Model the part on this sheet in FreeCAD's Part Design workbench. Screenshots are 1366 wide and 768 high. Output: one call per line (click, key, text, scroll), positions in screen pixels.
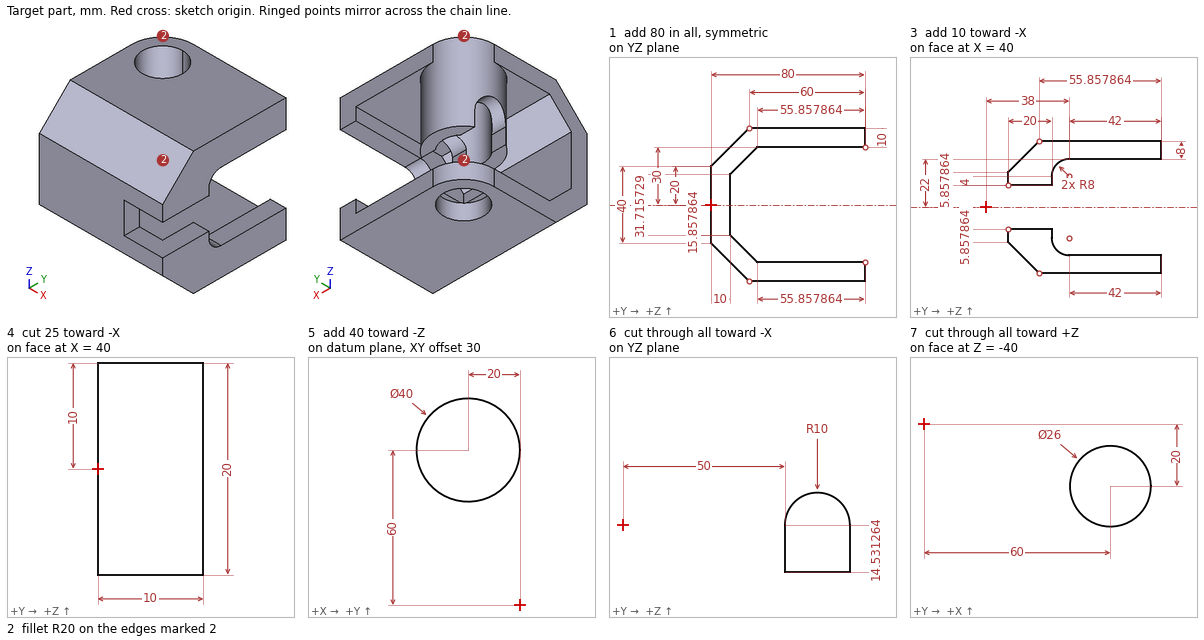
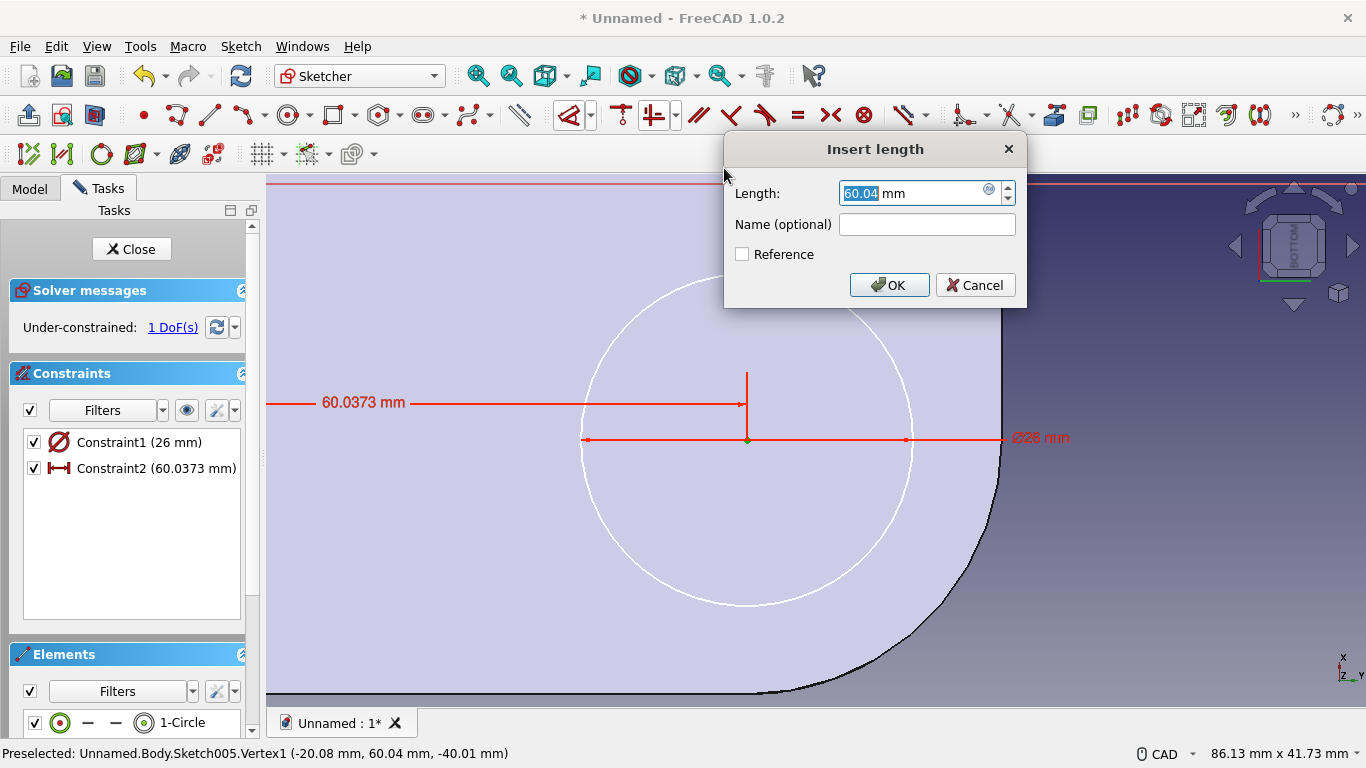
text(60)
key(Return)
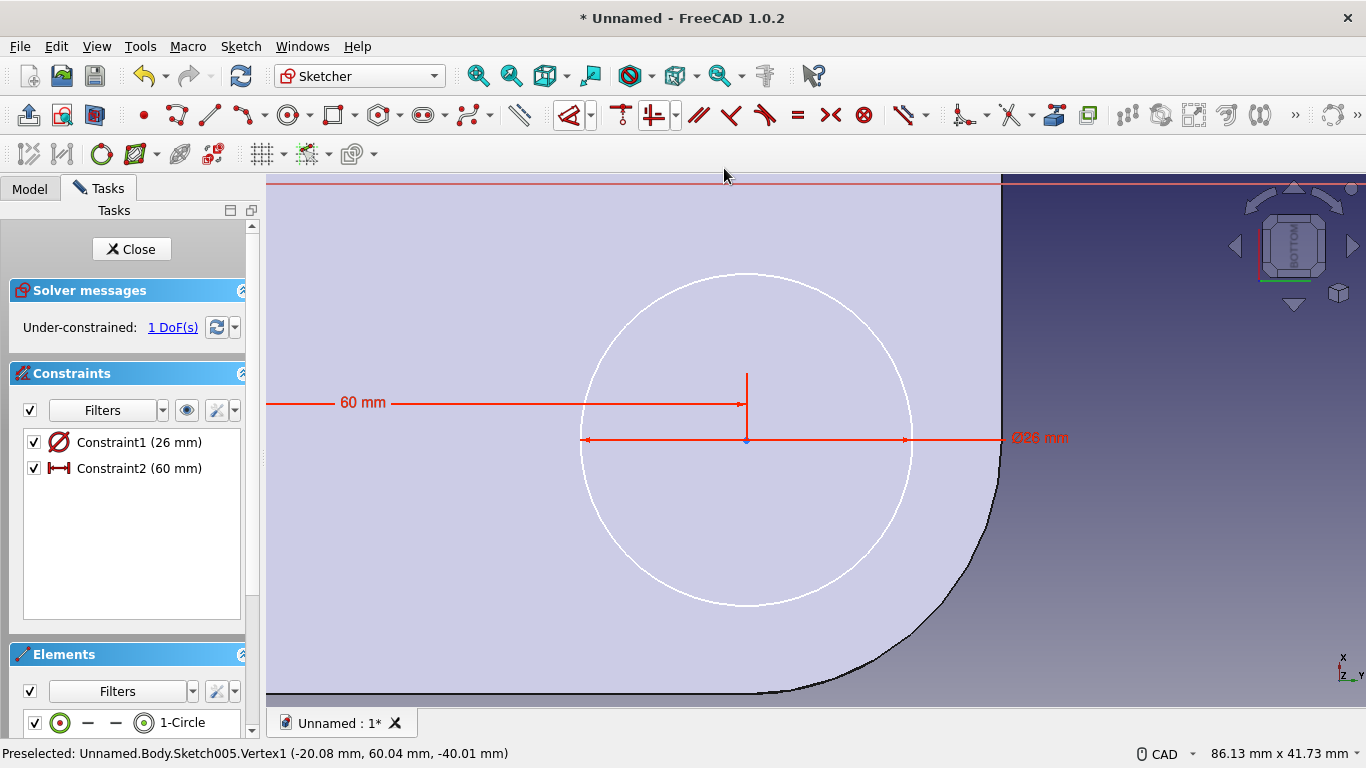
click(747, 440)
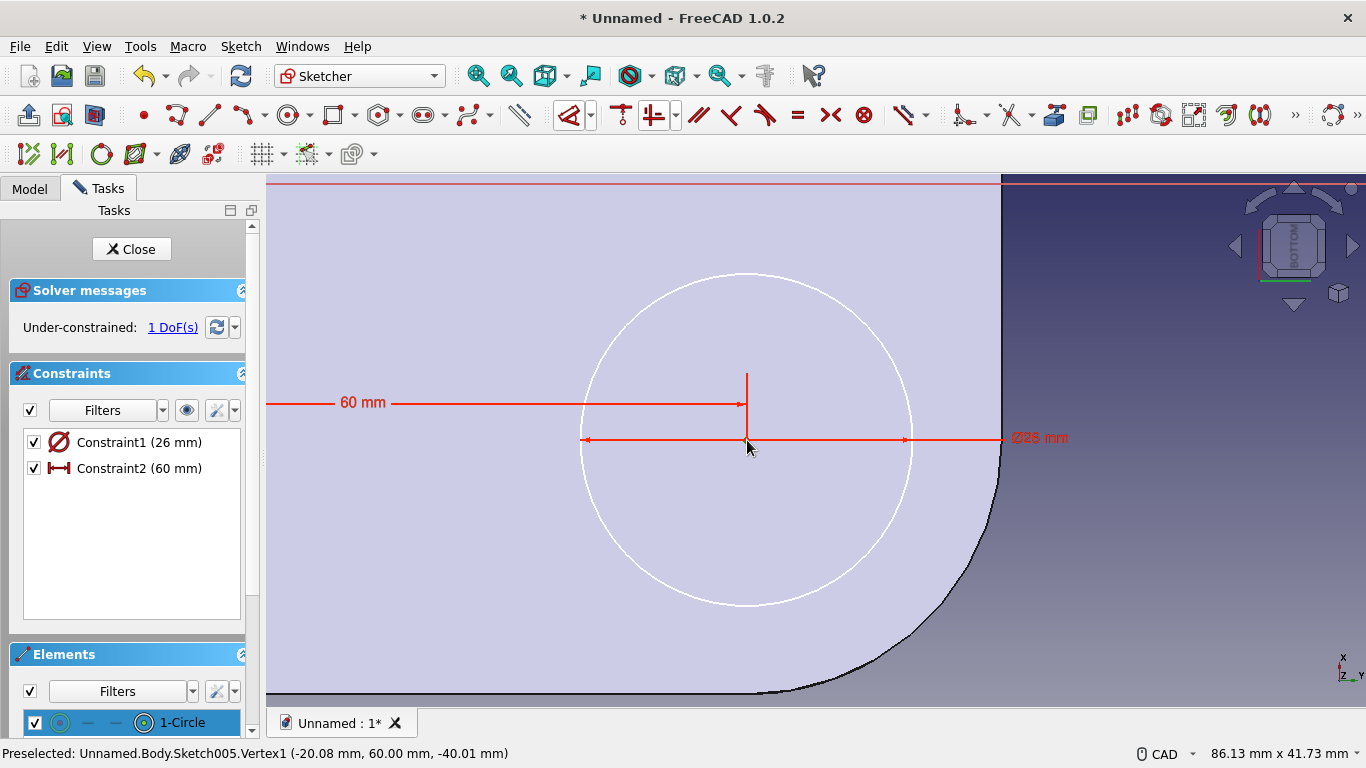
click(590, 116)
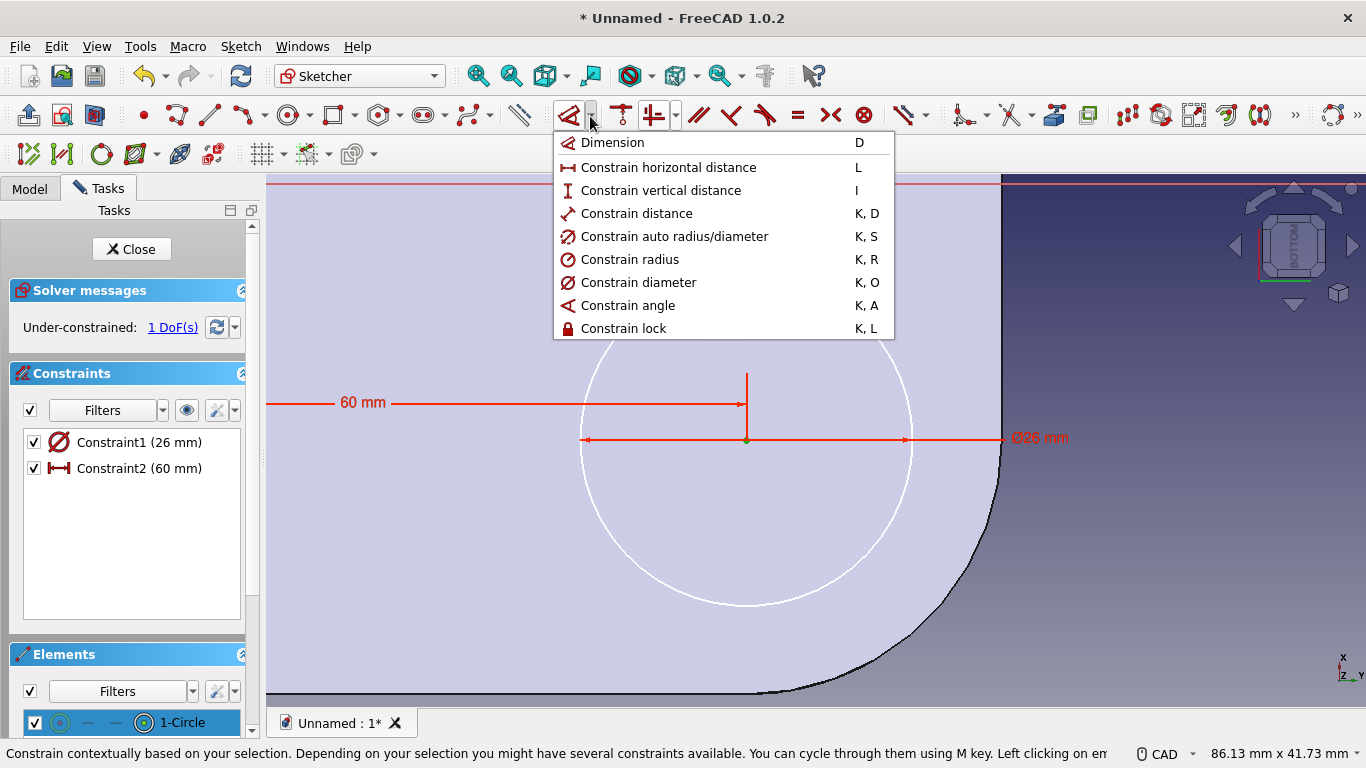
click(724, 190)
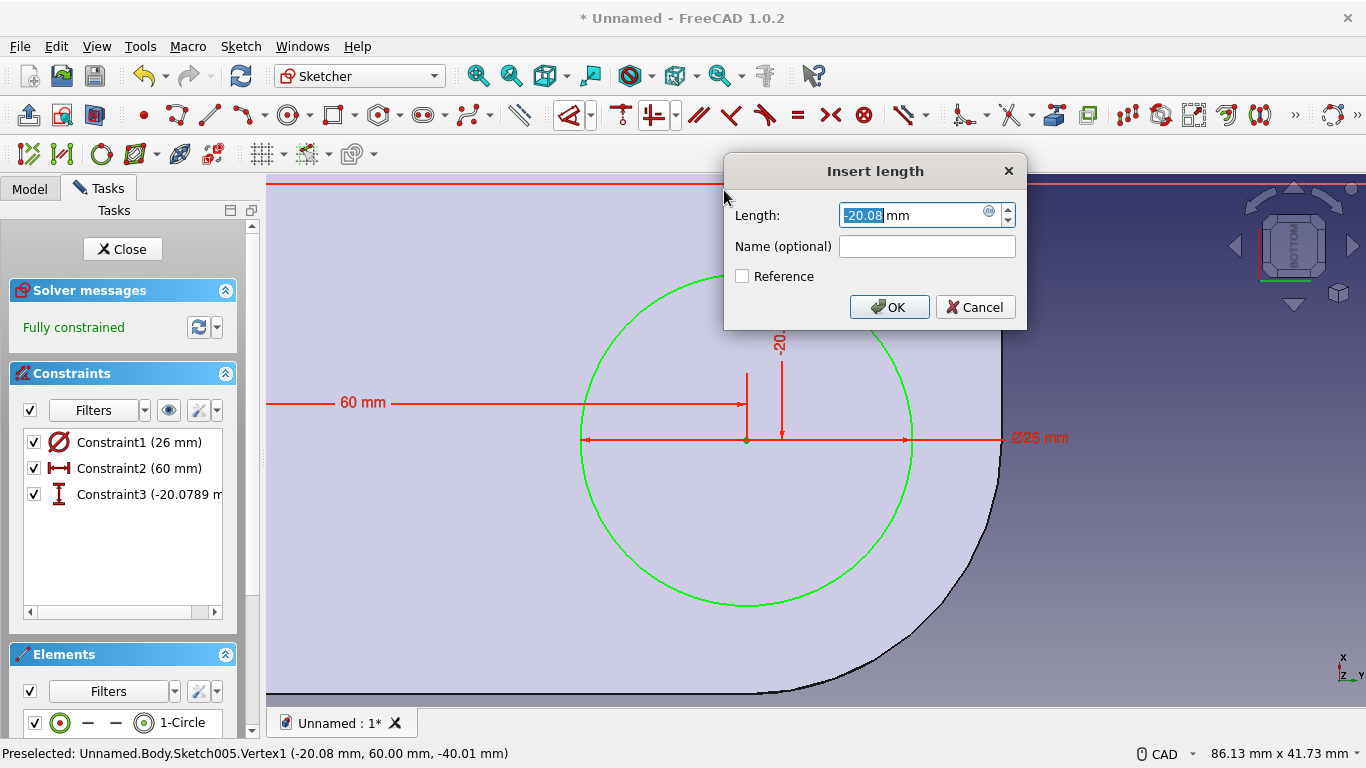
text(-20)
key(Return)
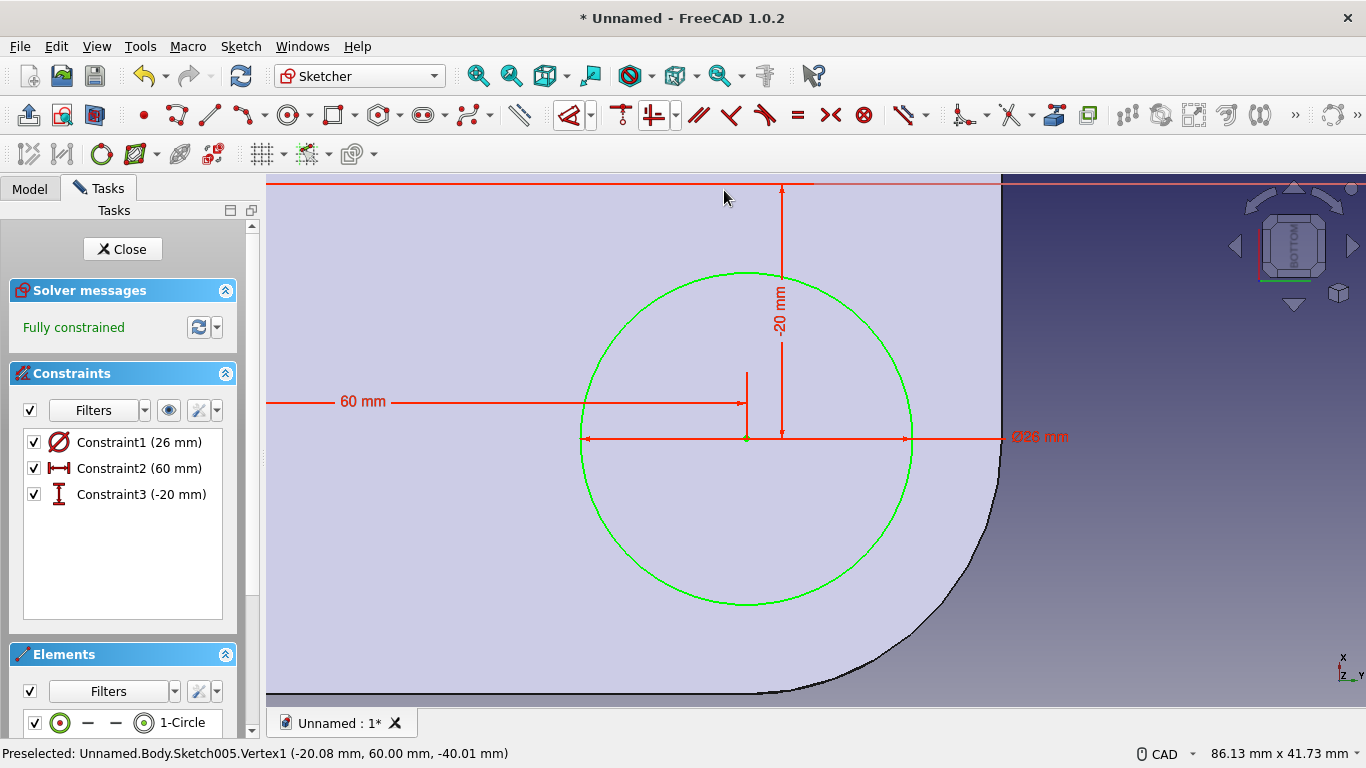
click(123, 249)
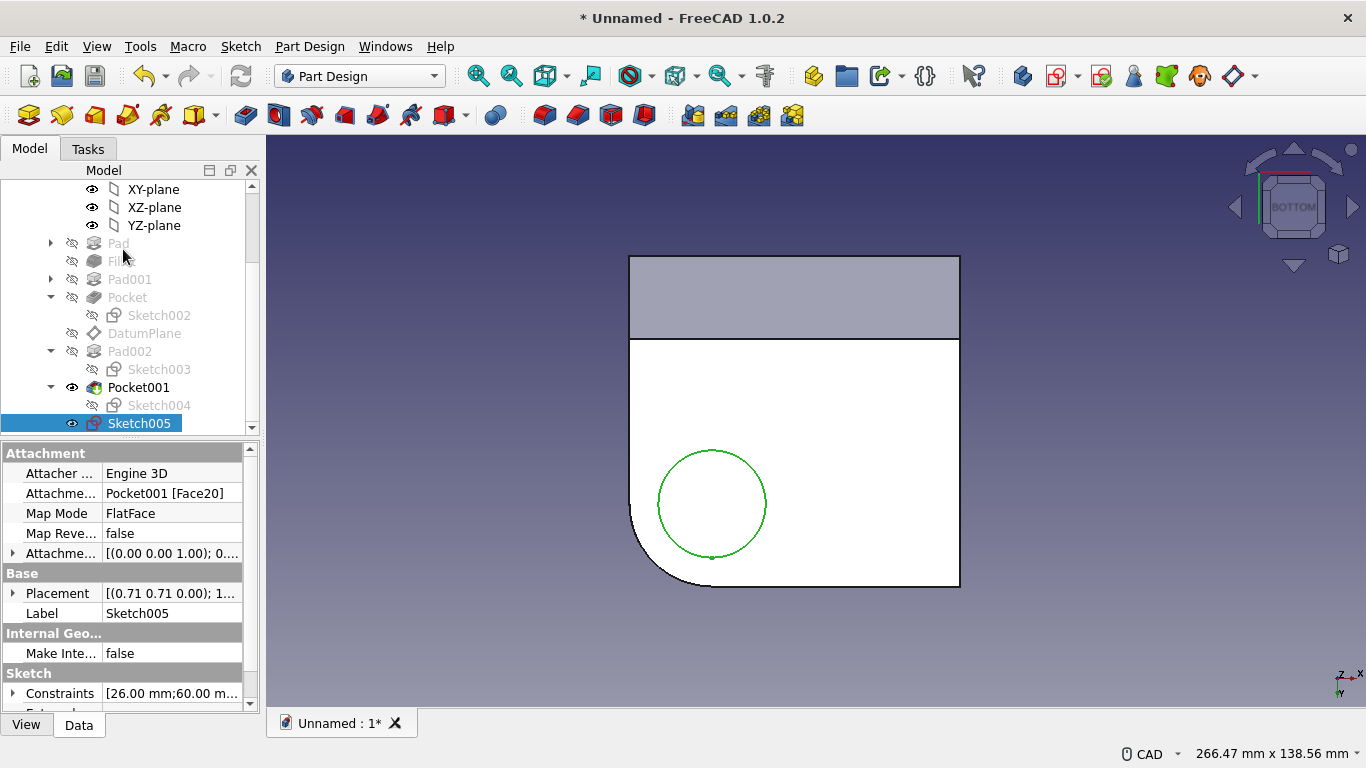
click(246, 116)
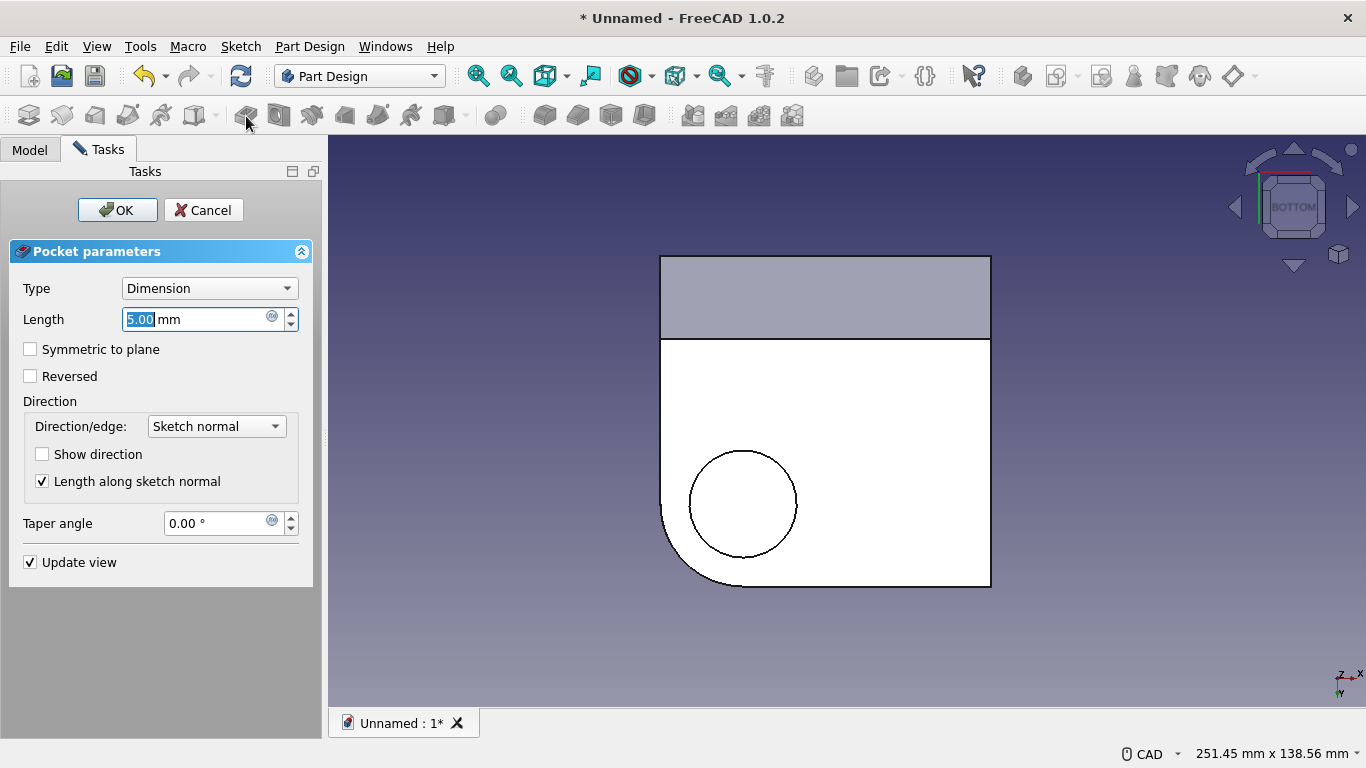
click(210, 288)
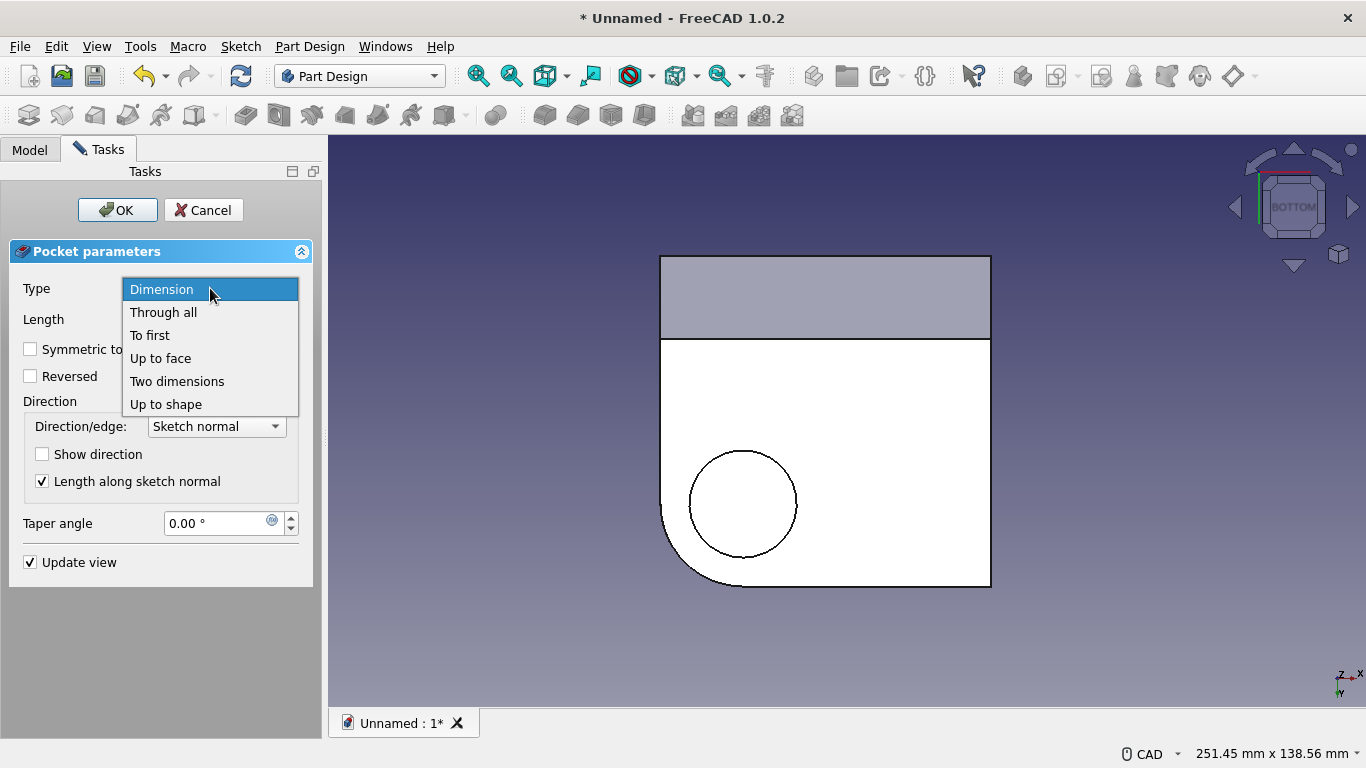
click(208, 312)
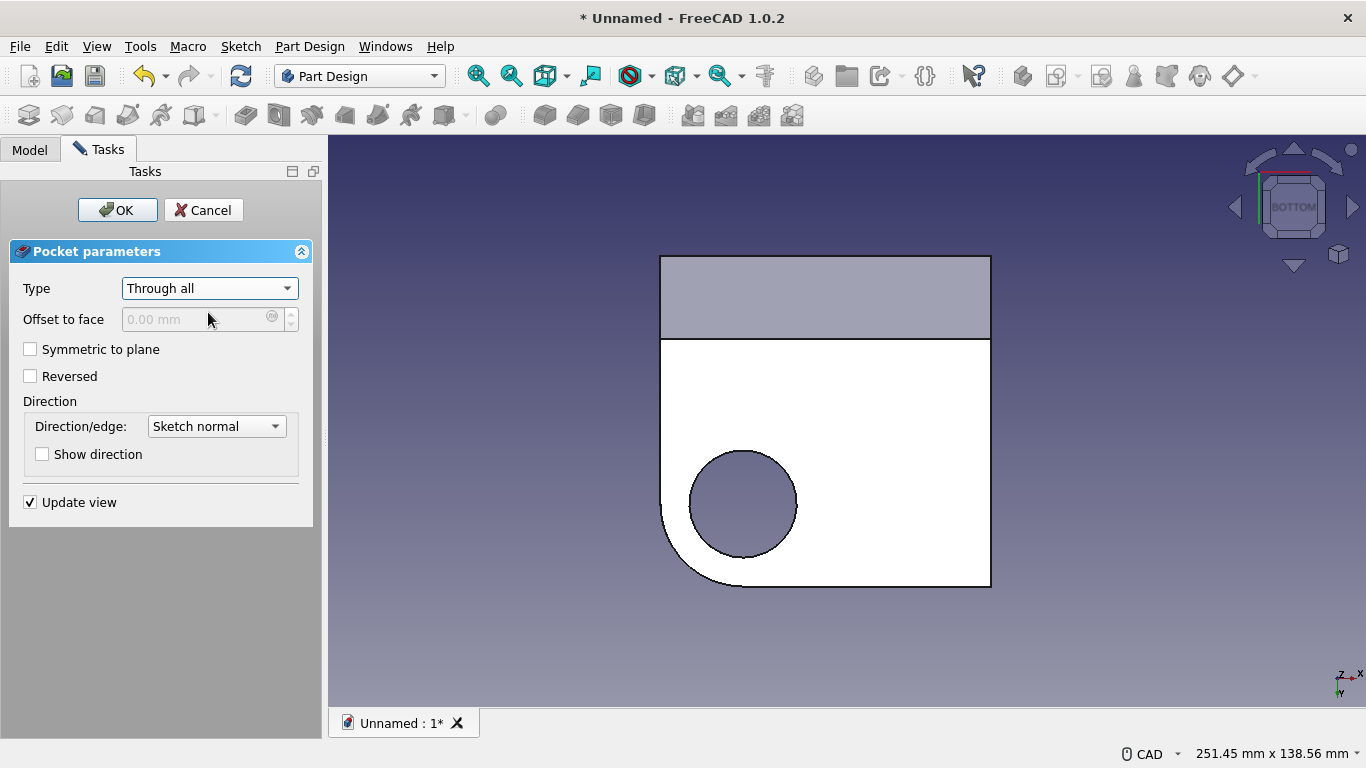
click(118, 210)